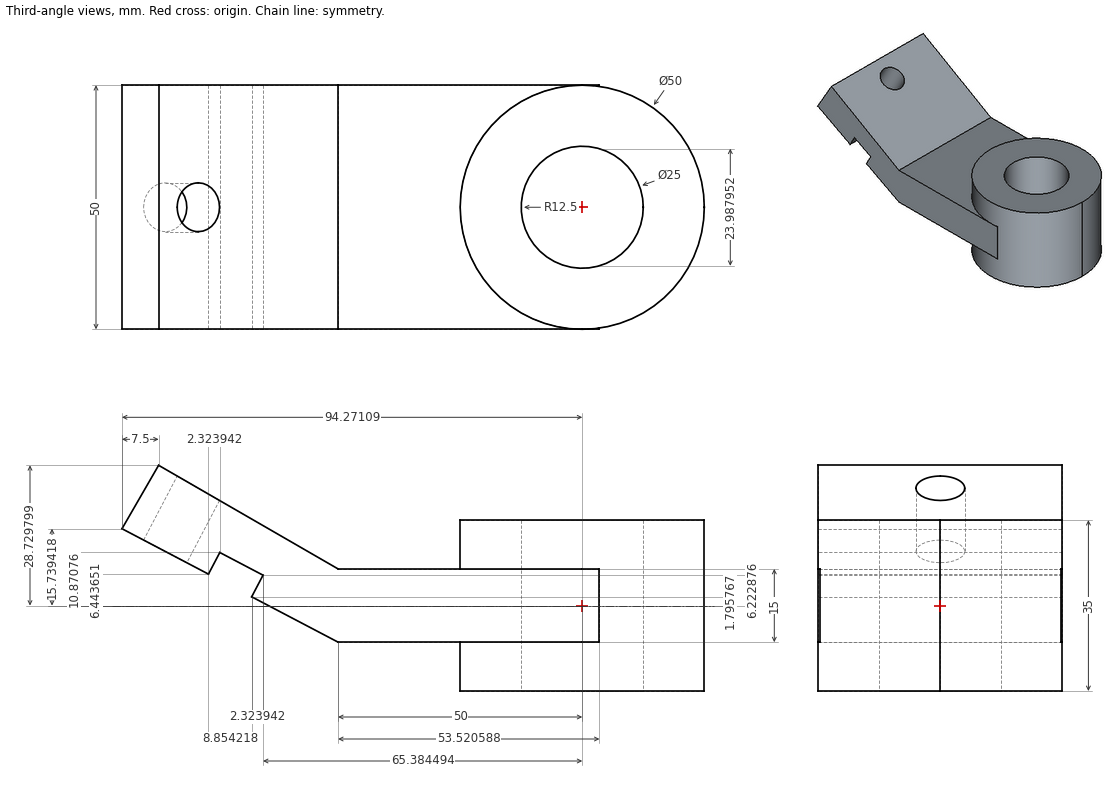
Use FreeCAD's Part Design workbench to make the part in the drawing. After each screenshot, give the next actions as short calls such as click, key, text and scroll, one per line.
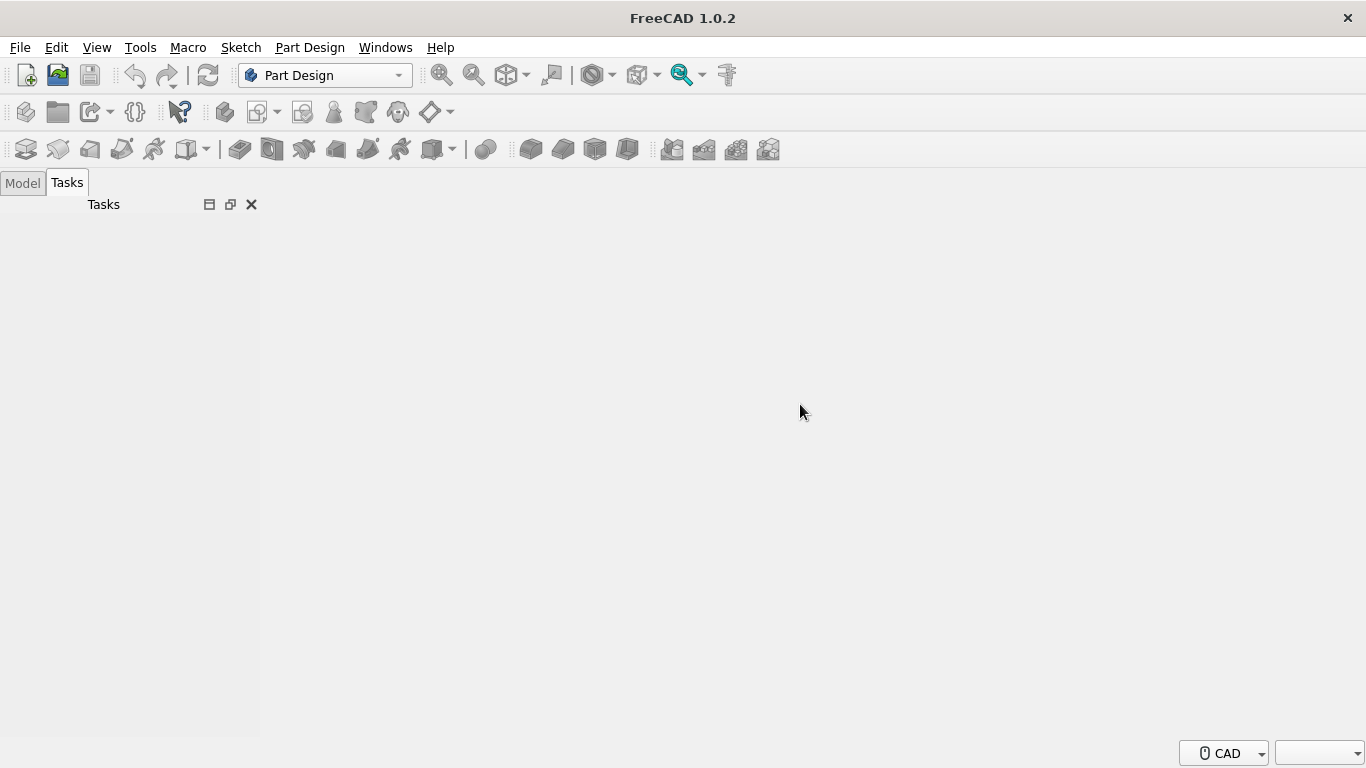
click(26, 76)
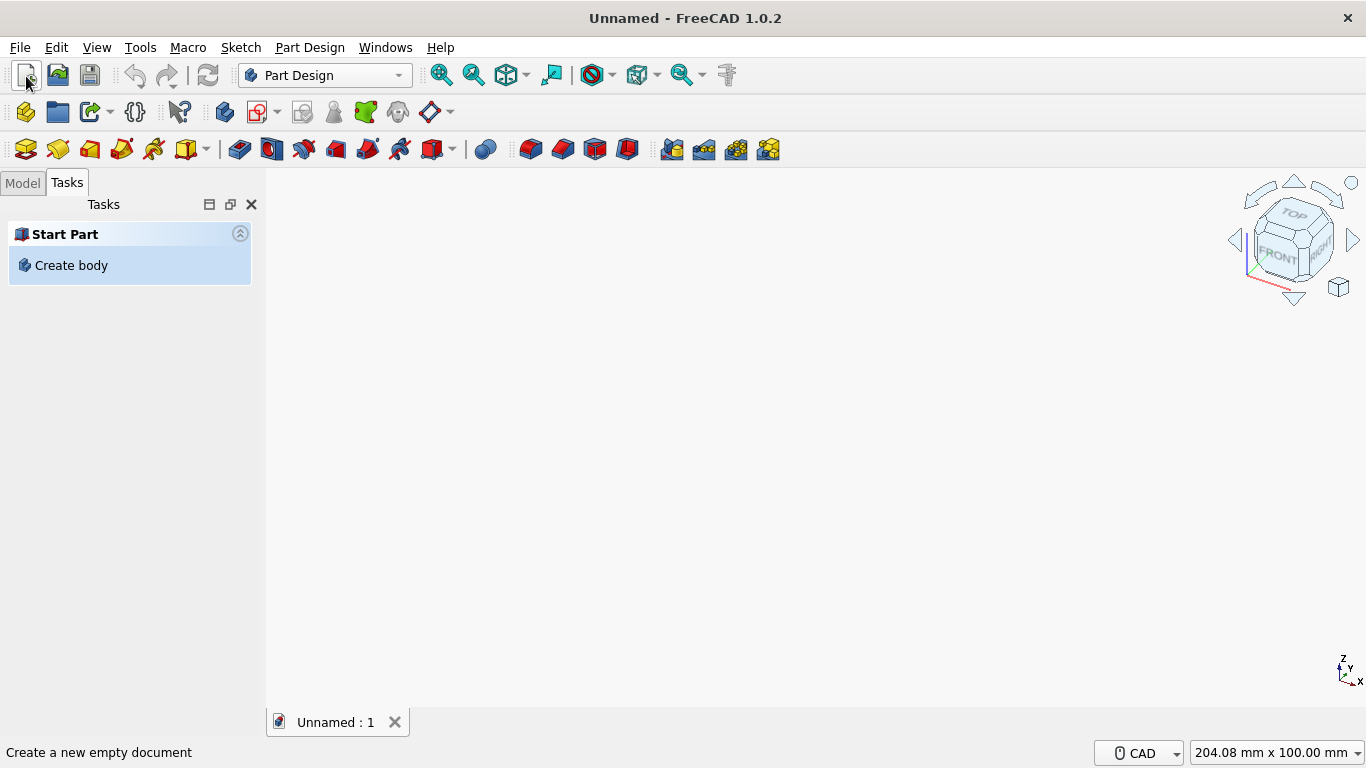
click(258, 112)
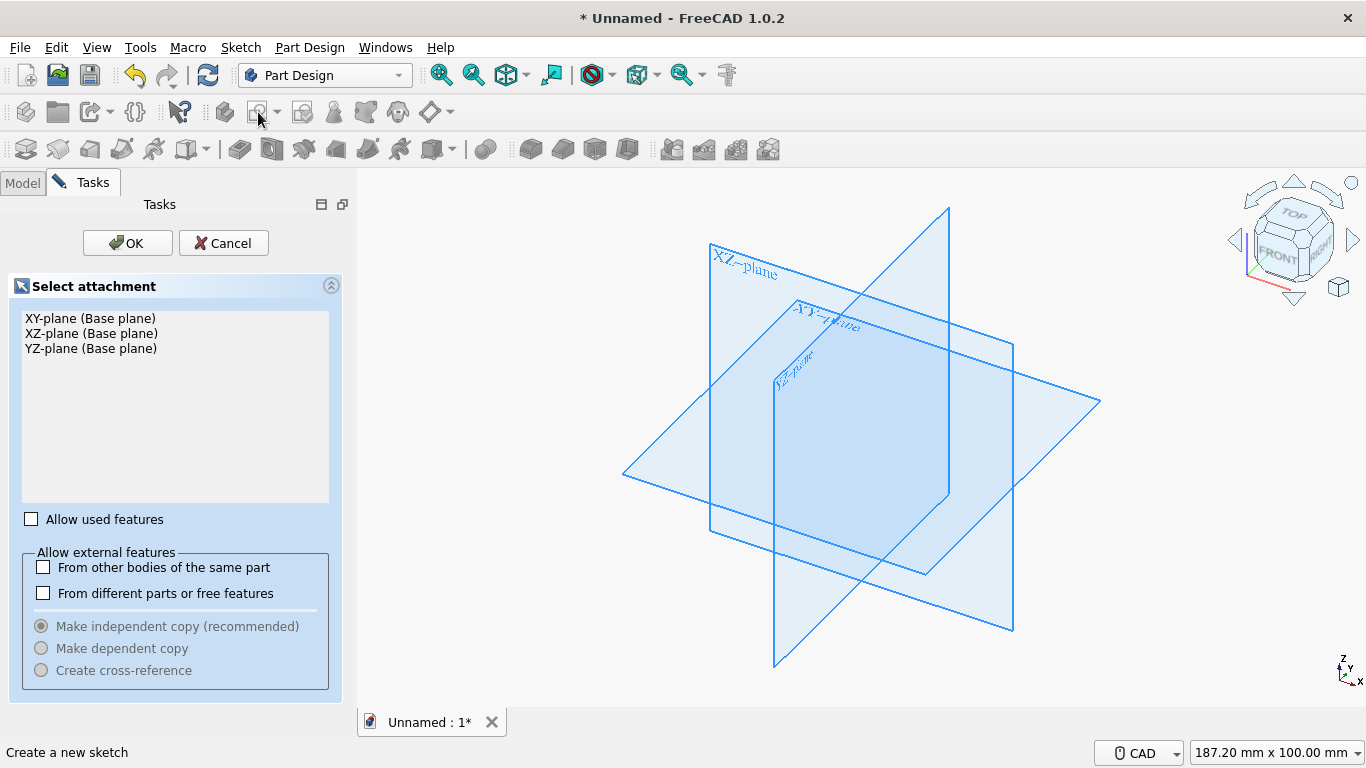
click(82, 318)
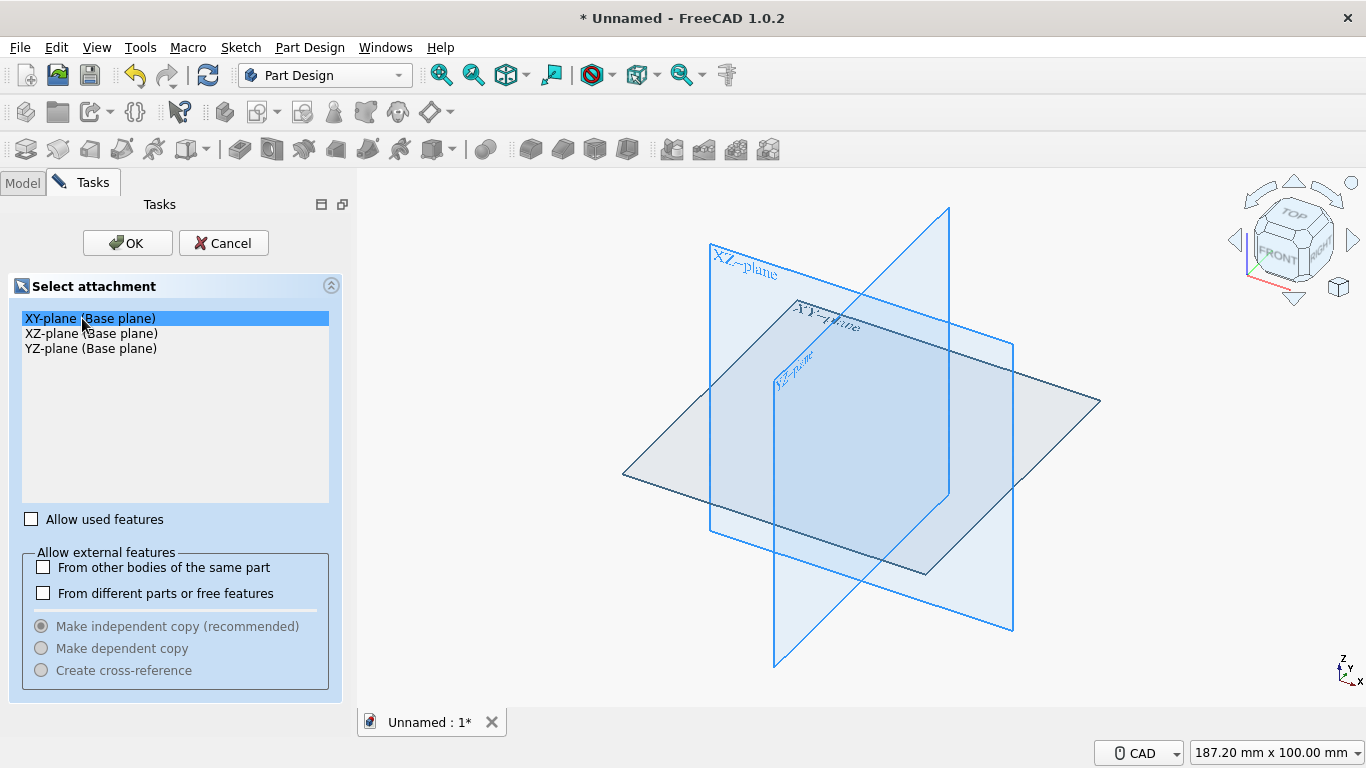
click(128, 243)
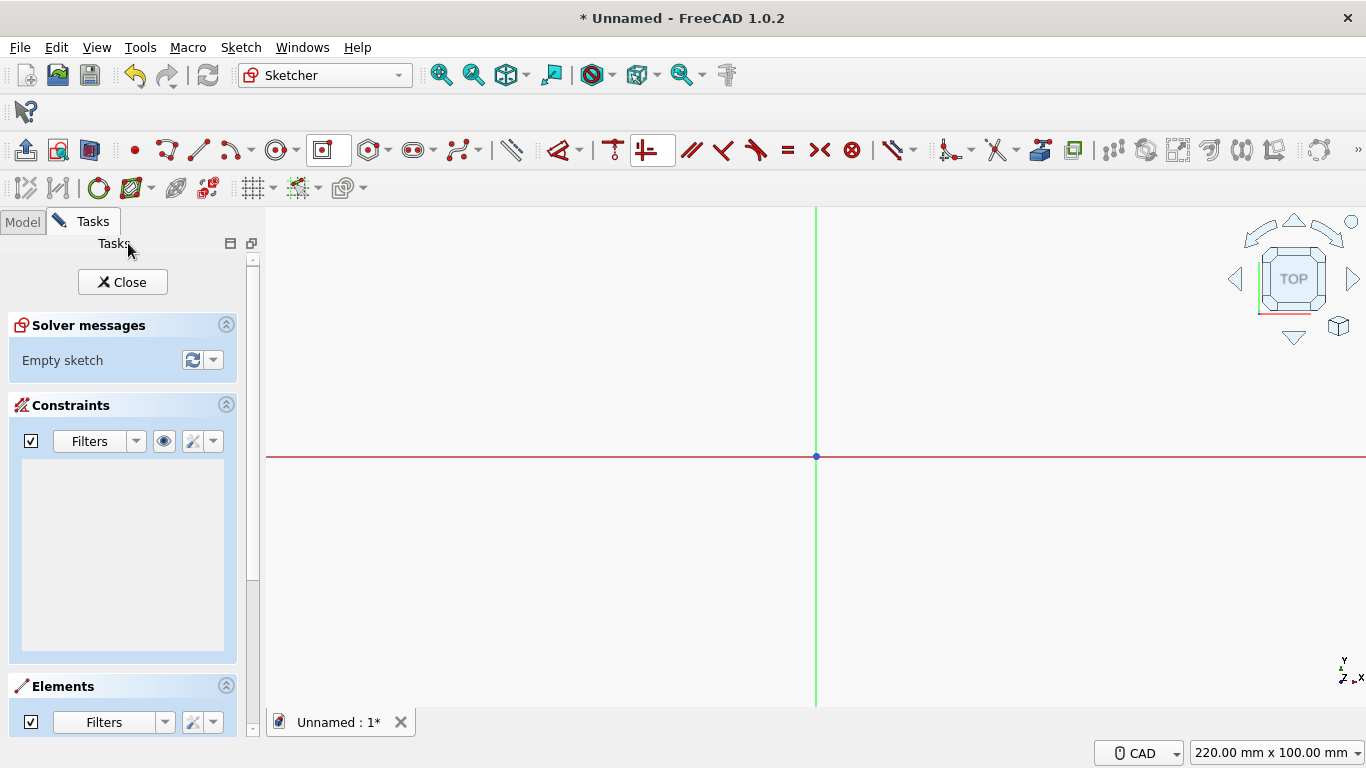
click(276, 150)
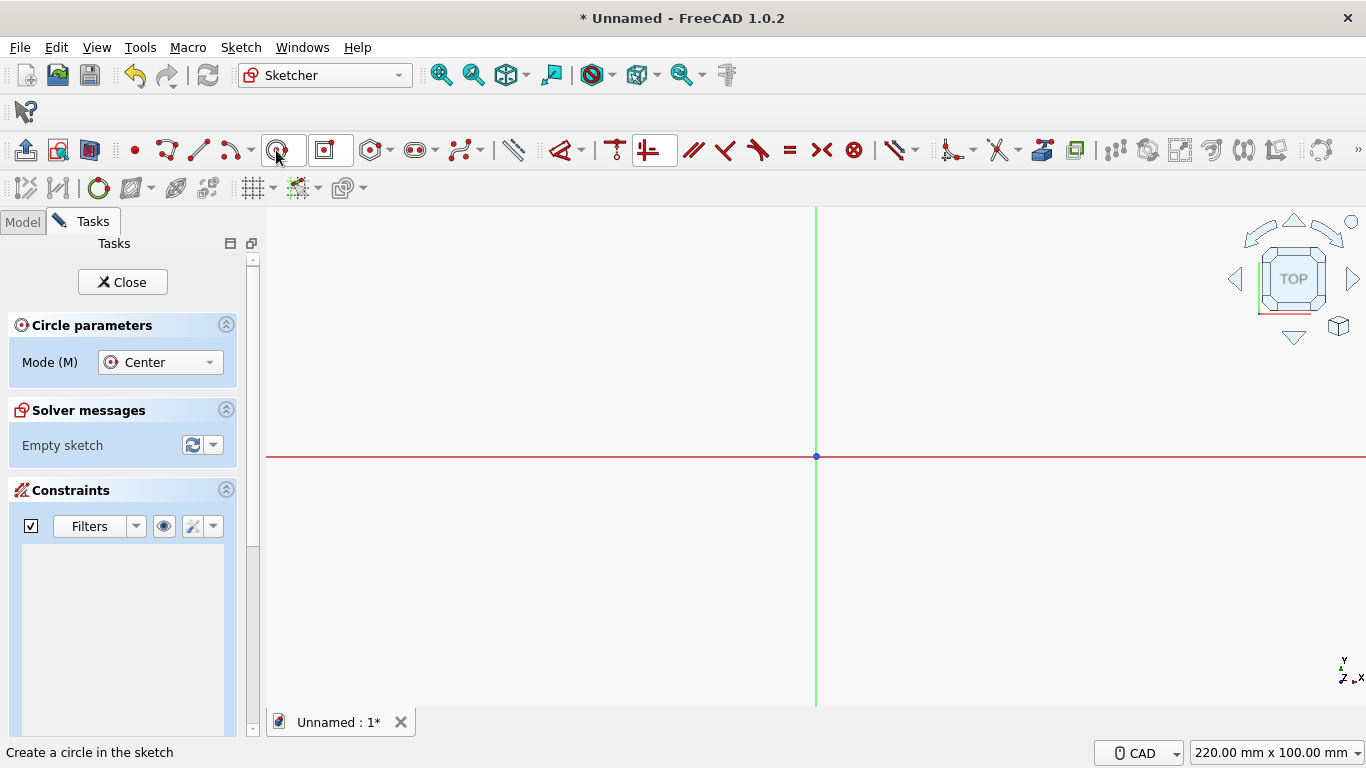
click(816, 457)
click(904, 369)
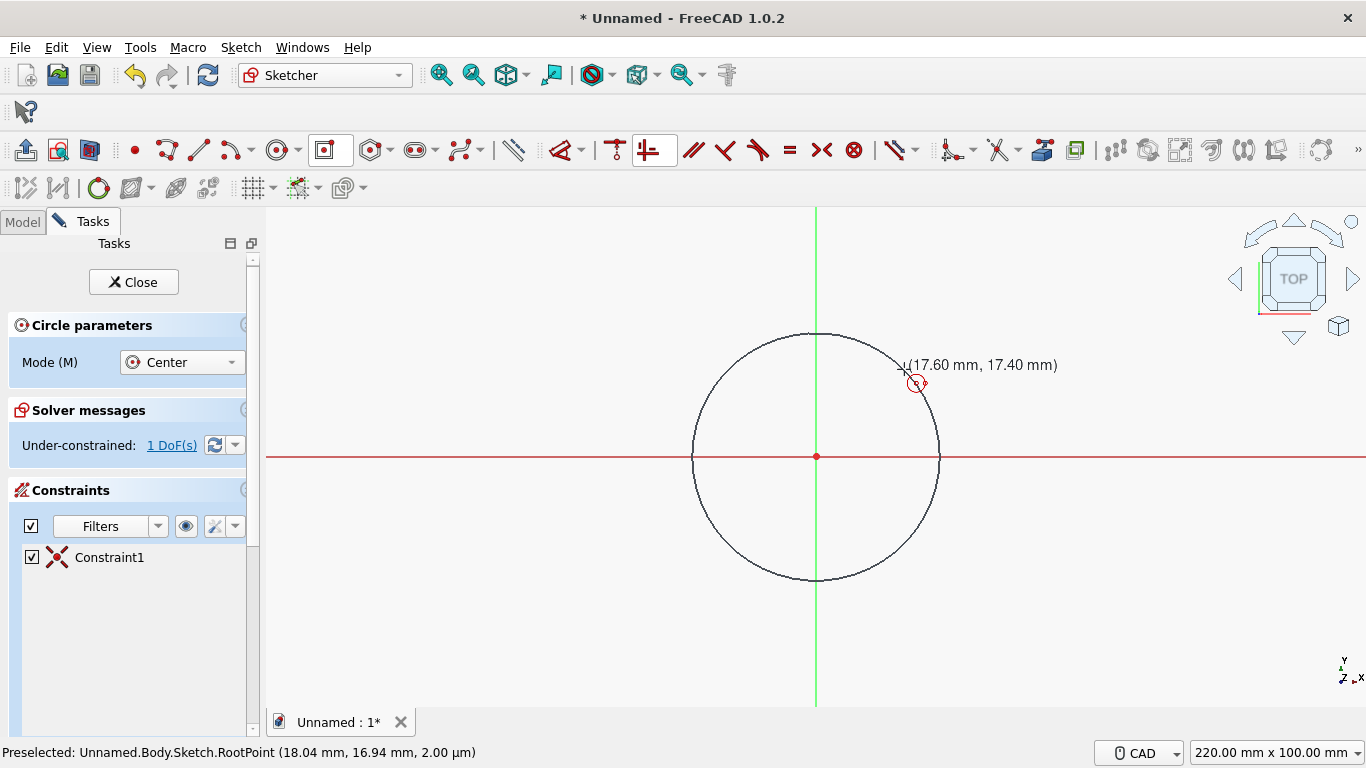
click(816, 457)
click(860, 413)
key(Escape)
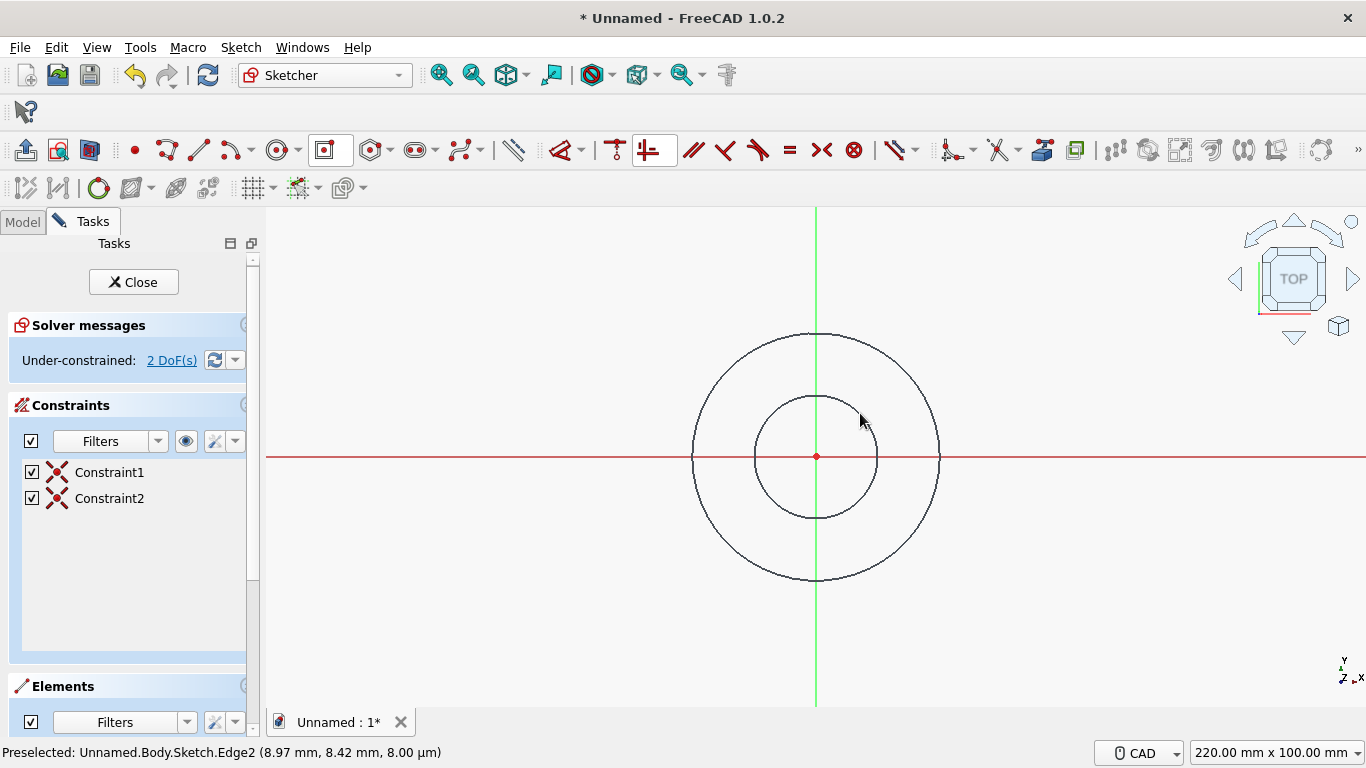
click(560, 150)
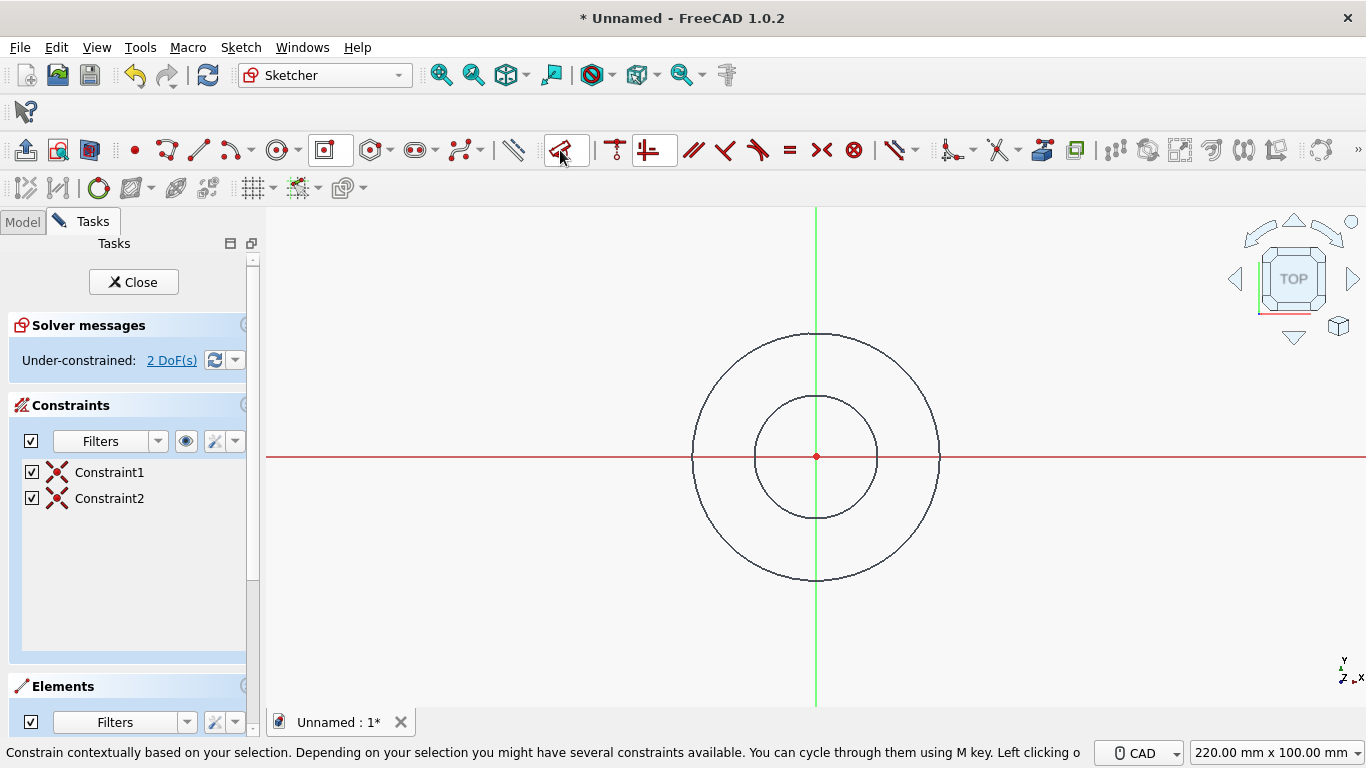
click(903, 369)
click(925, 346)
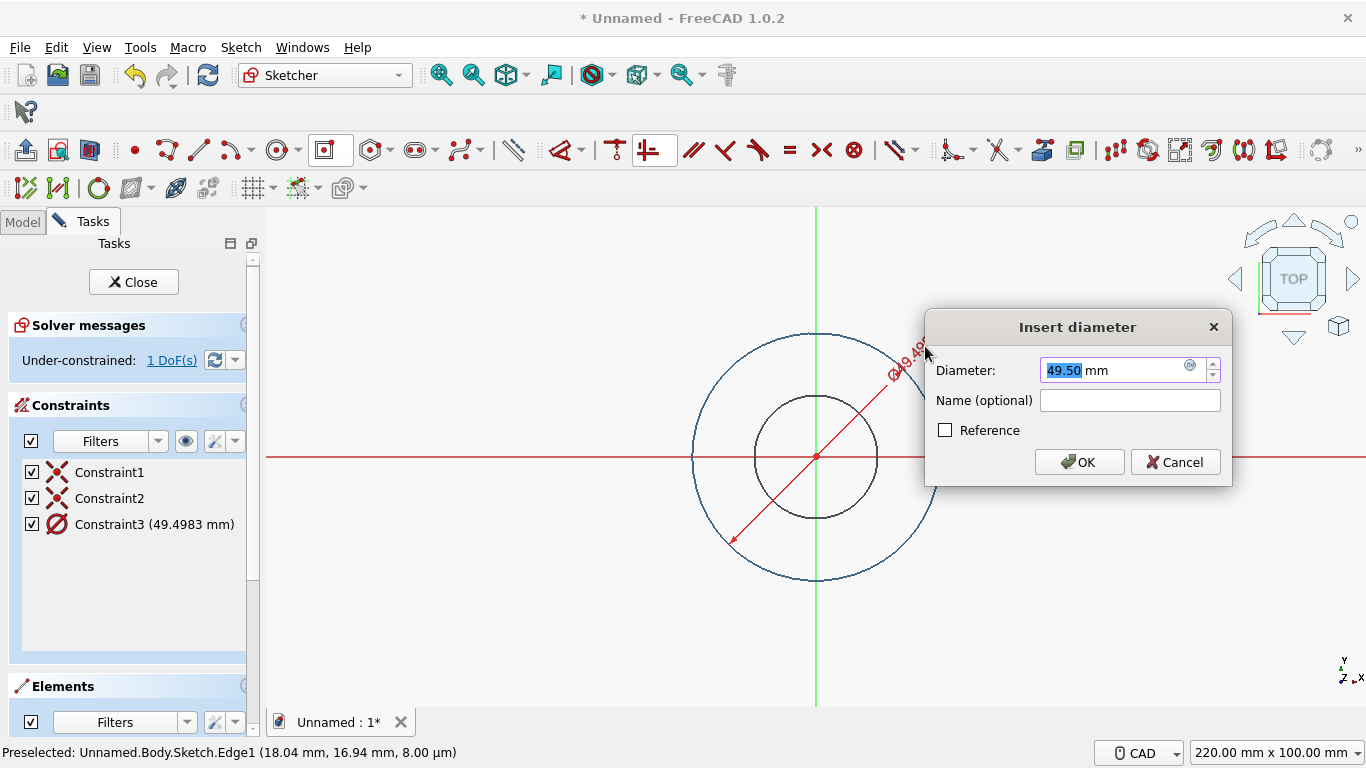
text(50)
key(Return)